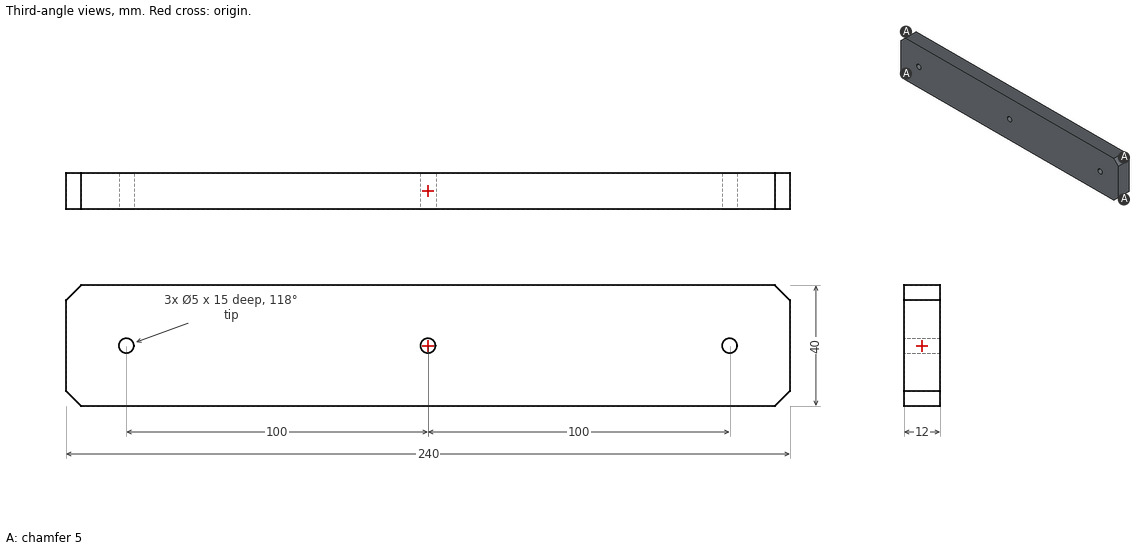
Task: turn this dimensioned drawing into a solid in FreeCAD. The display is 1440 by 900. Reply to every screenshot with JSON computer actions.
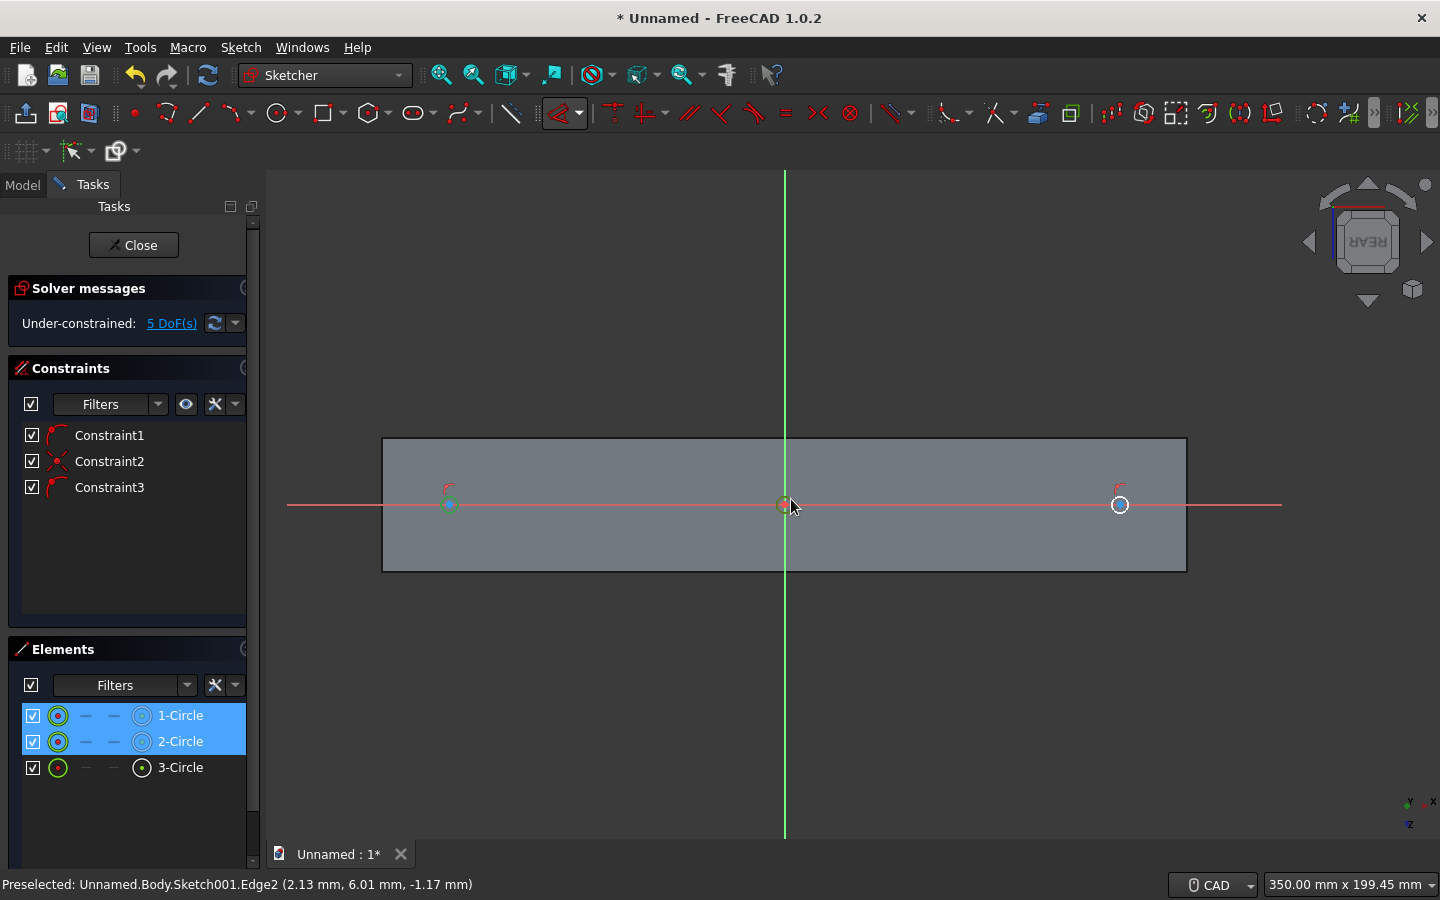
{"action": "scroll", "coordinate": [1126, 499], "scroll_direction": "up", "scroll_amount": 5}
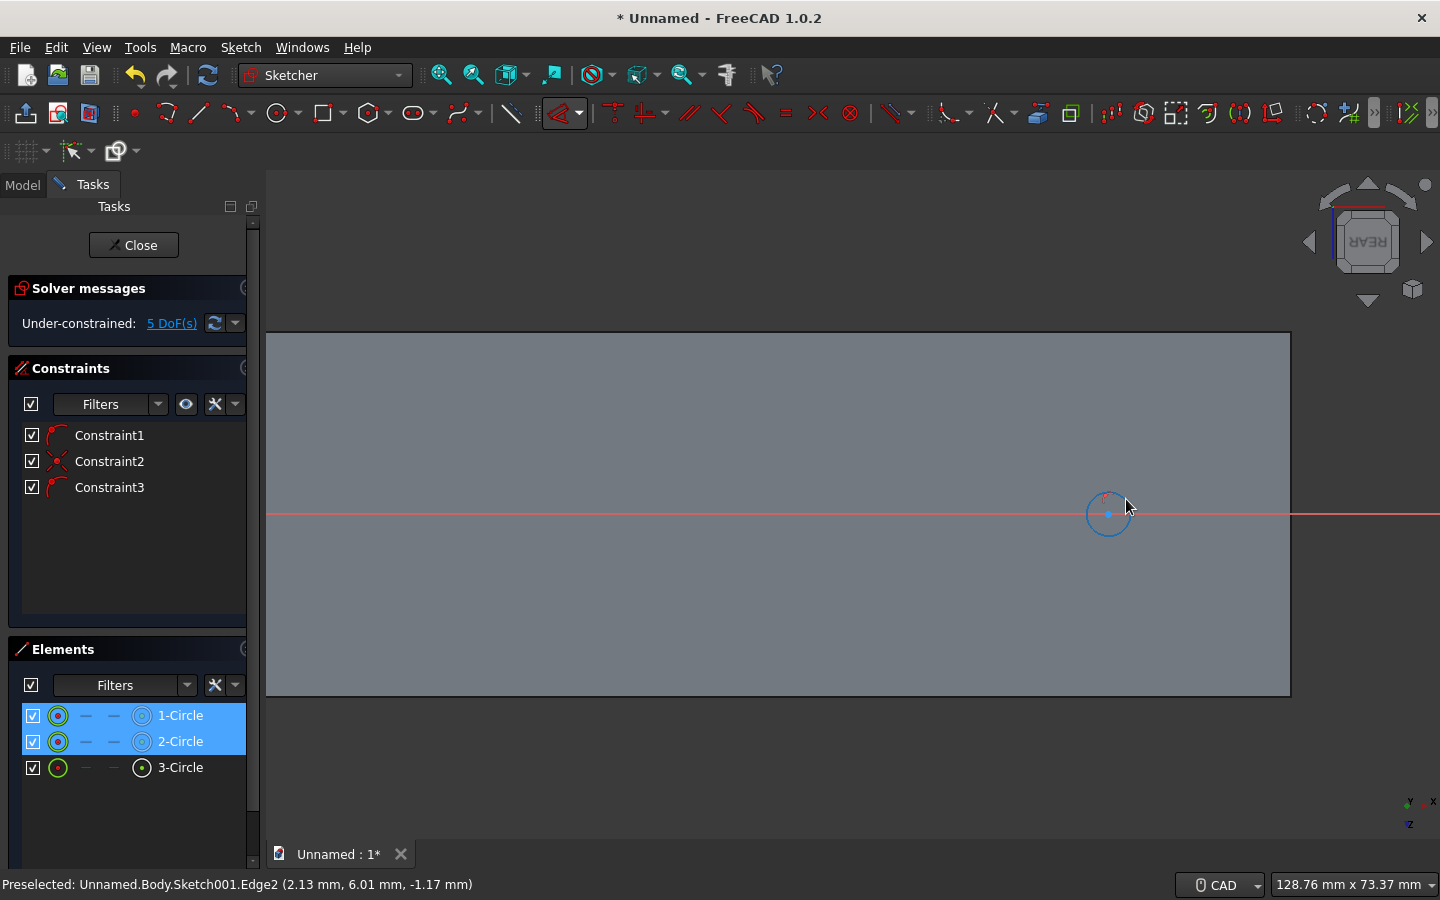
{"action": "left_click", "coordinate": [1124, 499]}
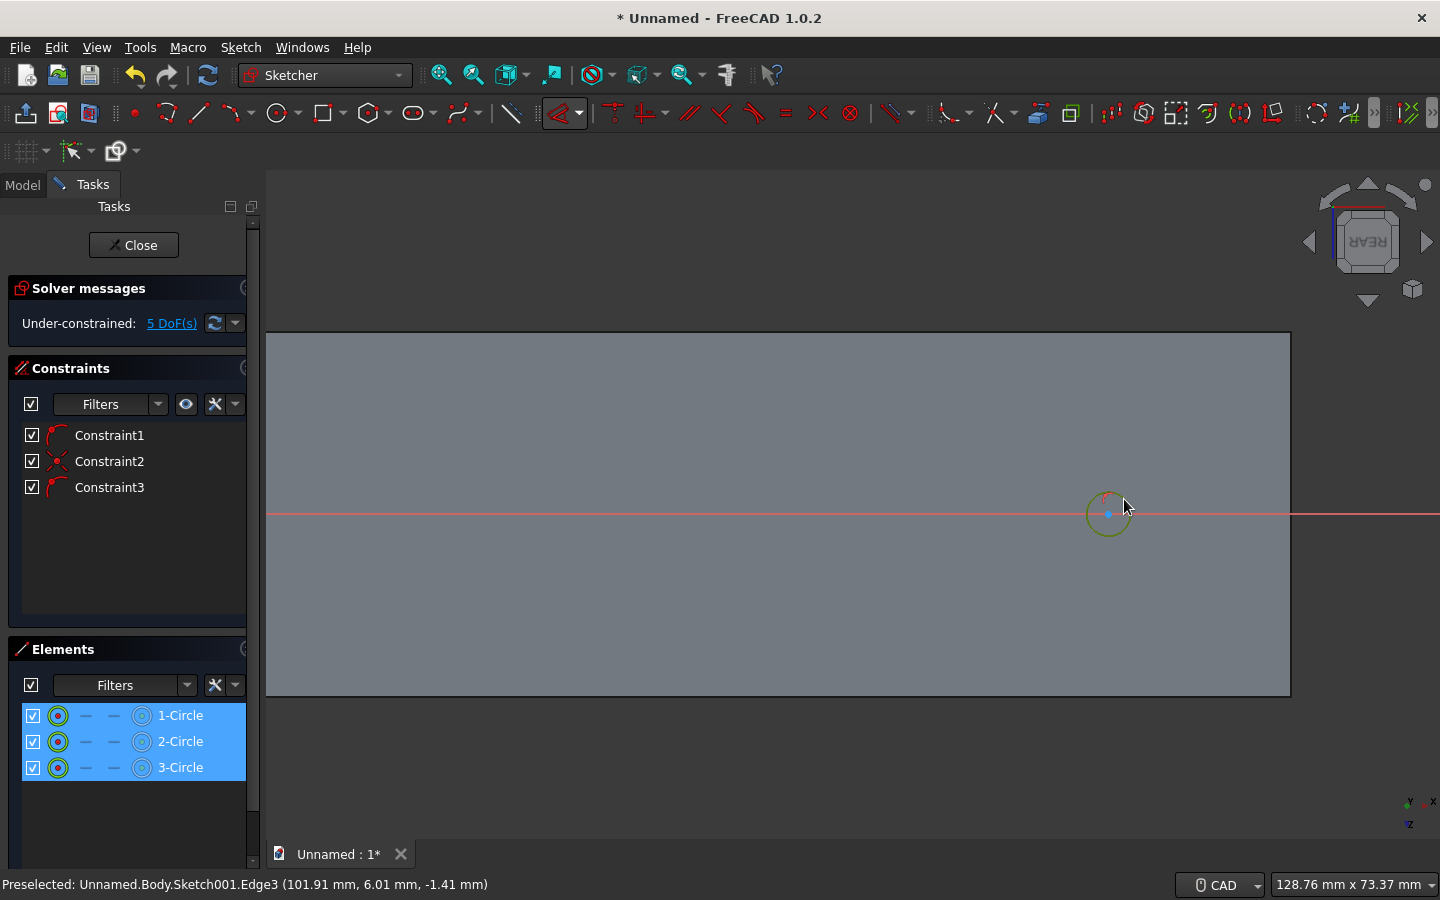
{"action": "left_click", "coordinate": [786, 114]}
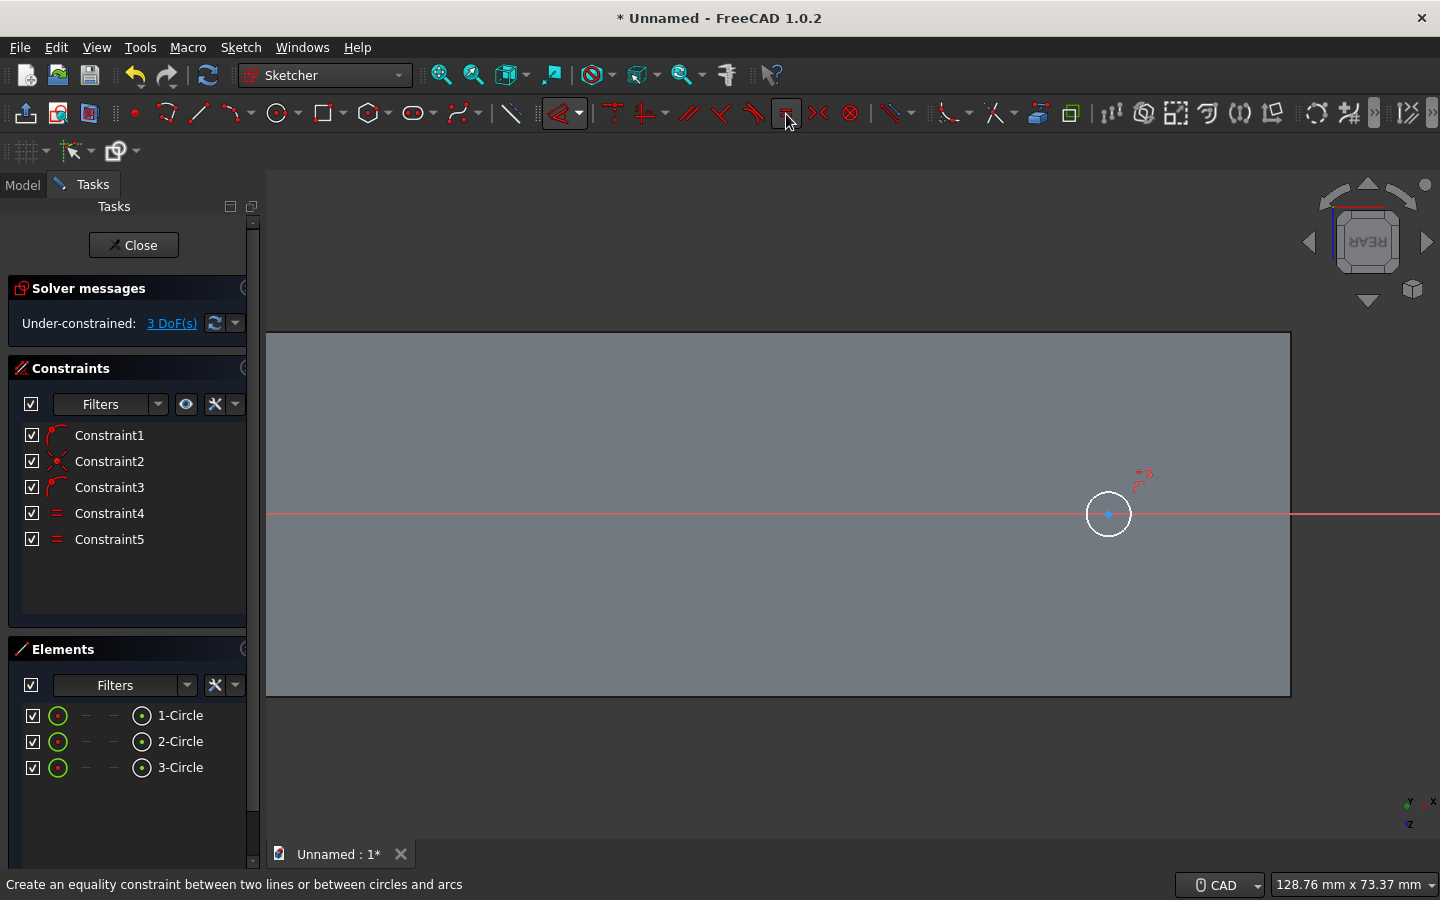
{"action": "scroll", "coordinate": [1126, 499], "scroll_direction": "down", "scroll_amount": 5}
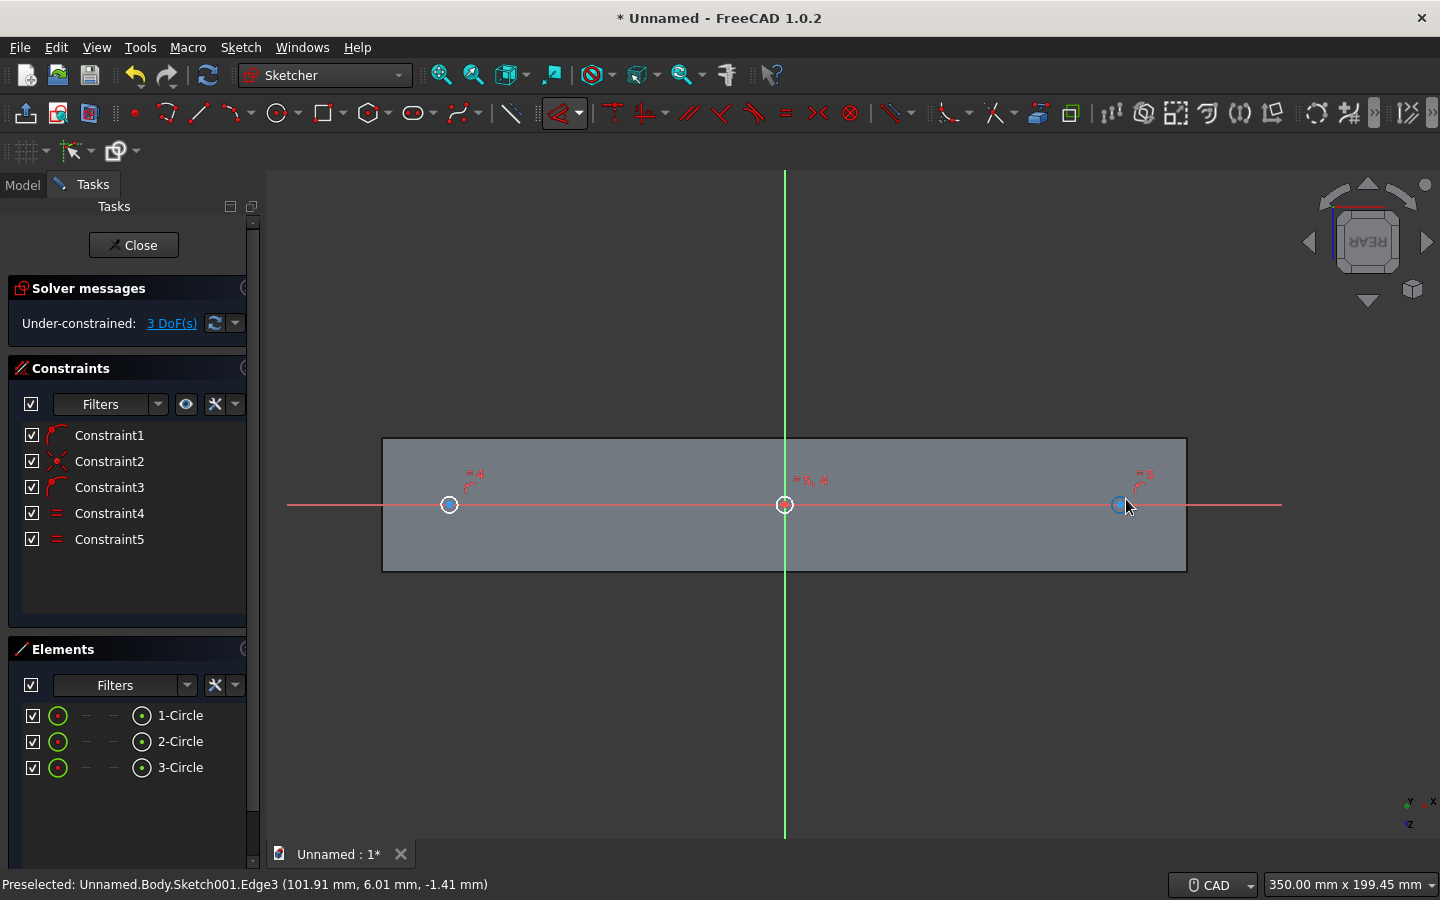
{"action": "scroll", "coordinate": [455, 499], "scroll_direction": "up", "scroll_amount": 5}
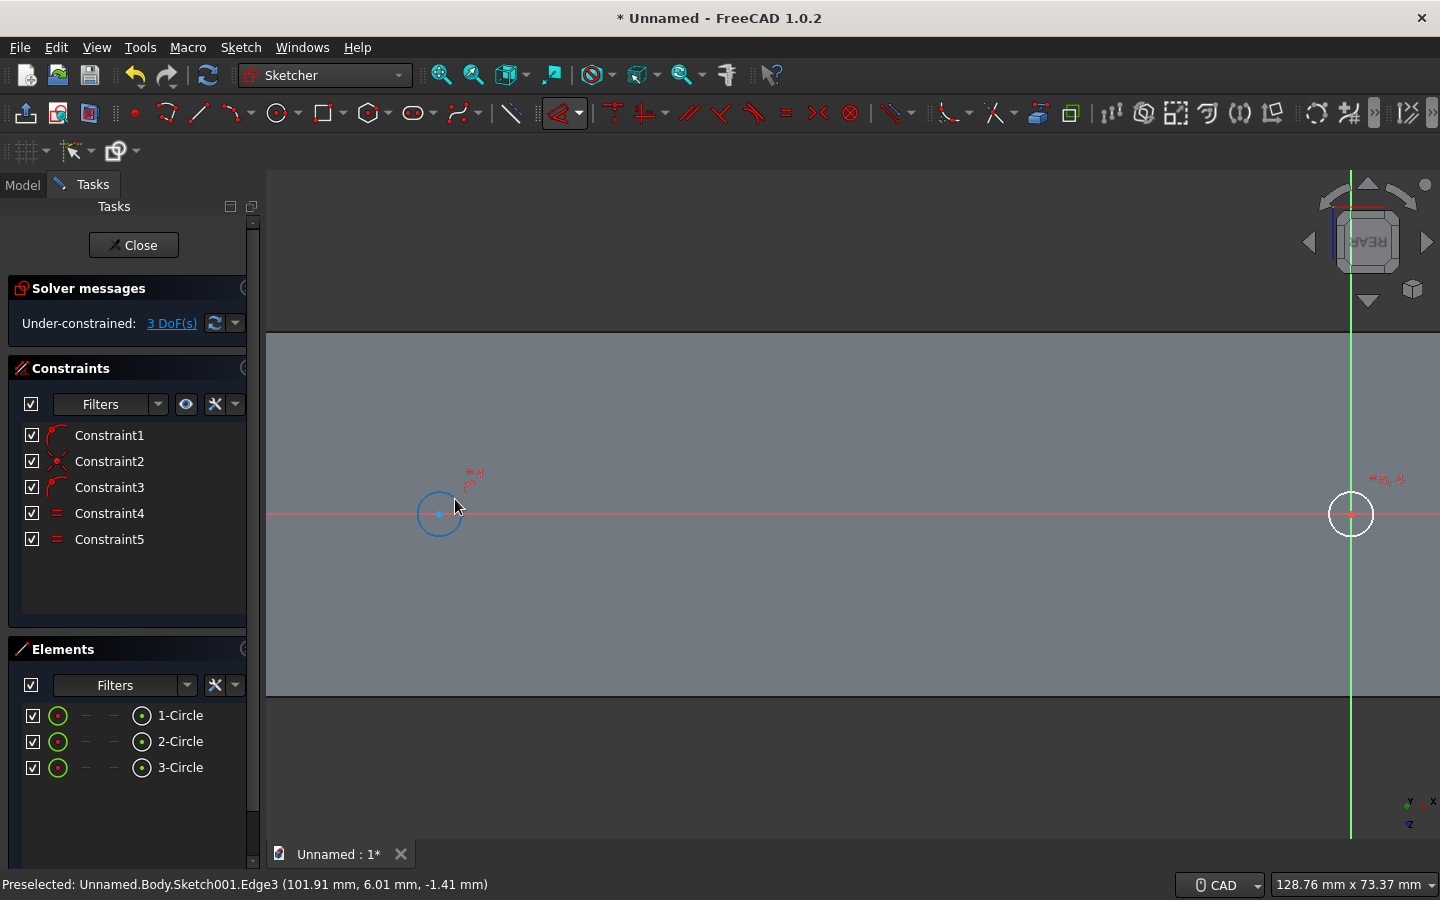
{"action": "left_click", "coordinate": [455, 499]}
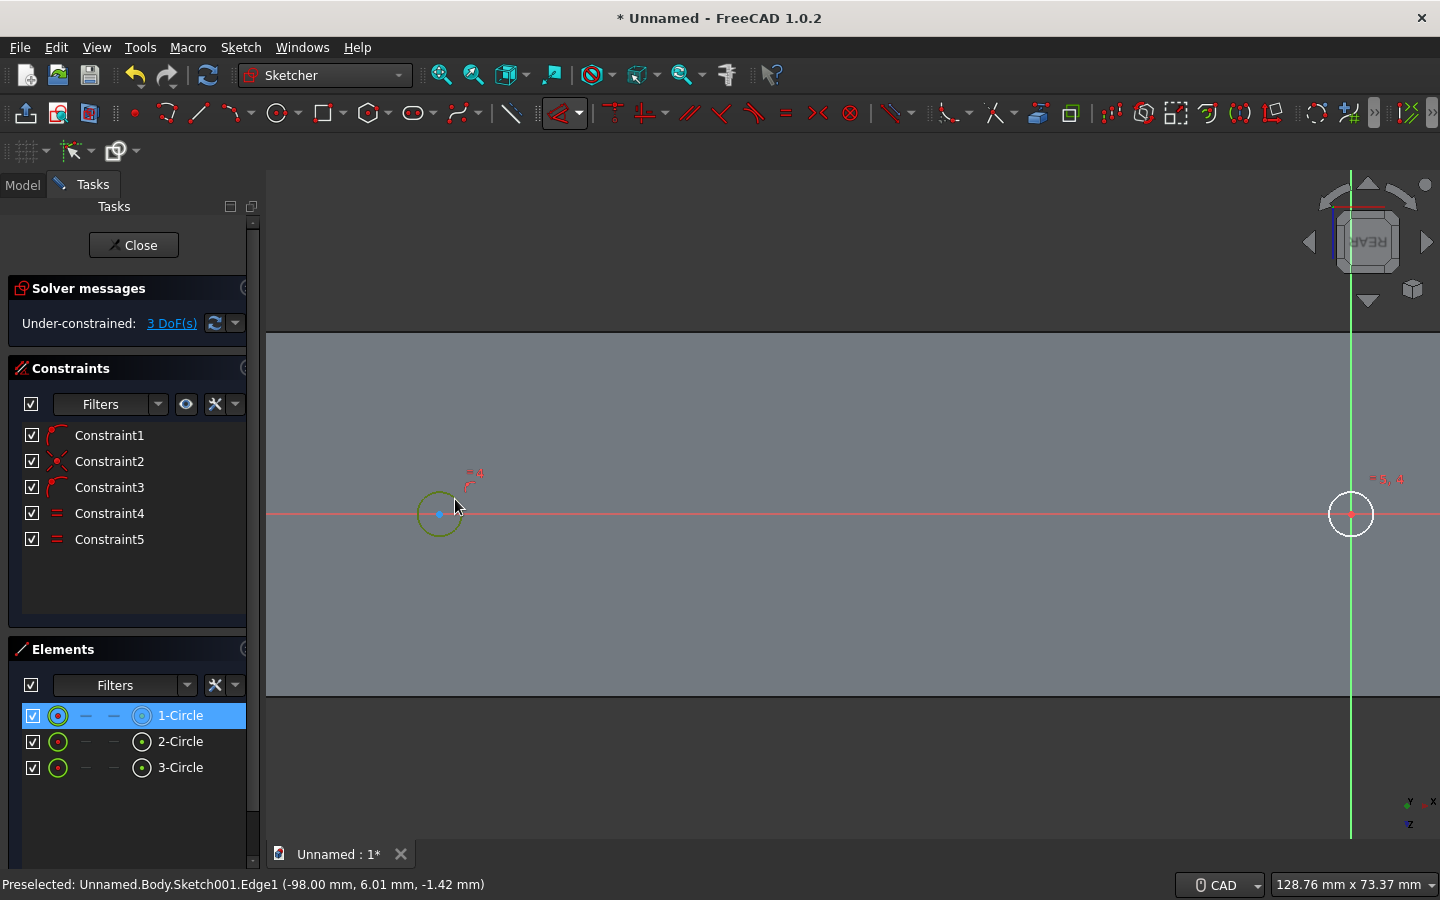
{"action": "left_click", "coordinate": [582, 114]}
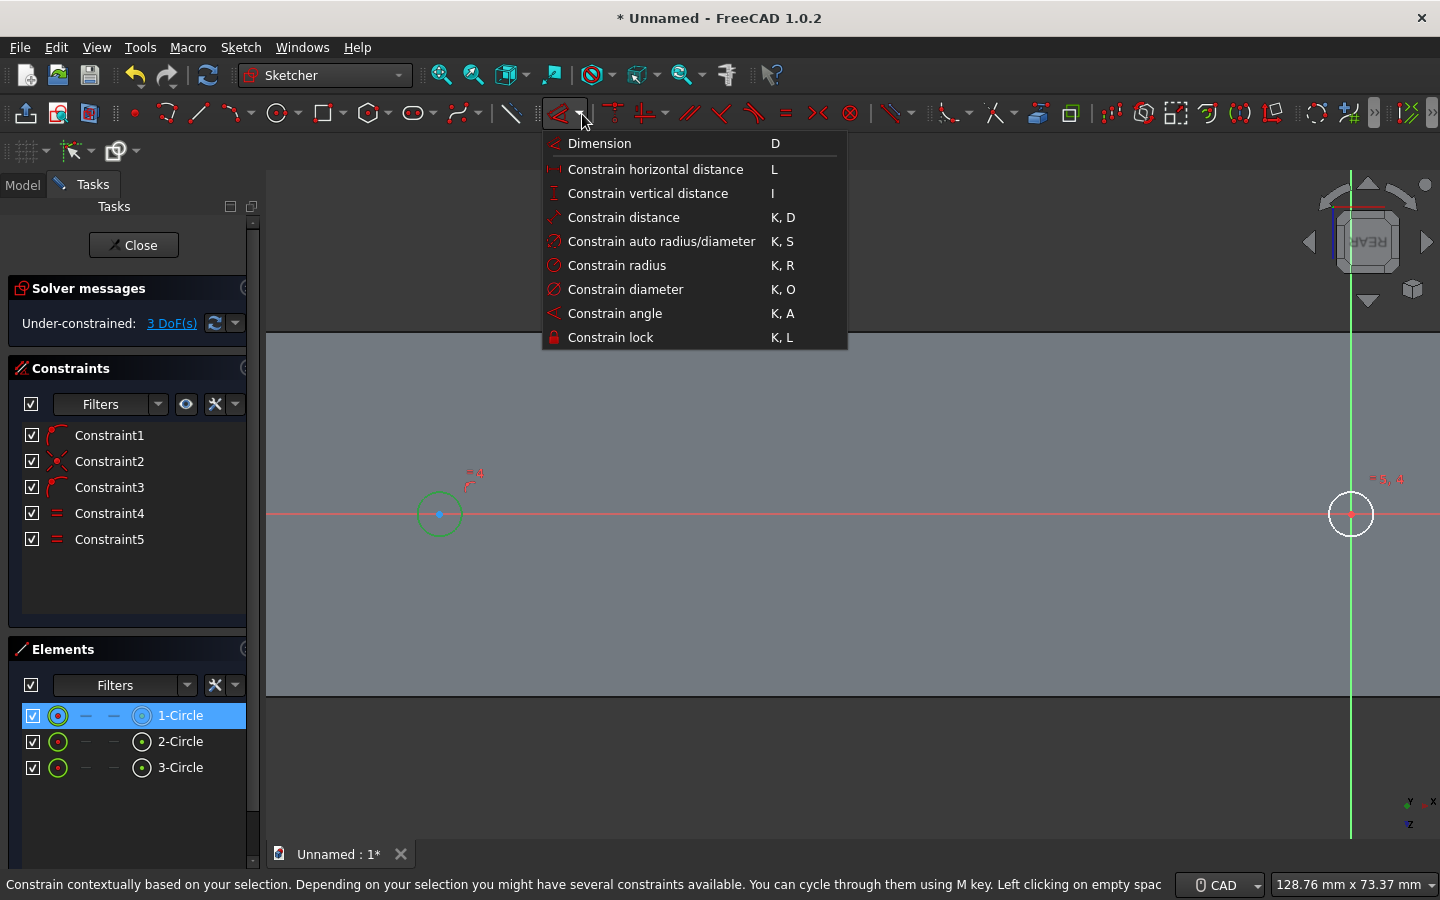
{"action": "left_click", "coordinate": [695, 289]}